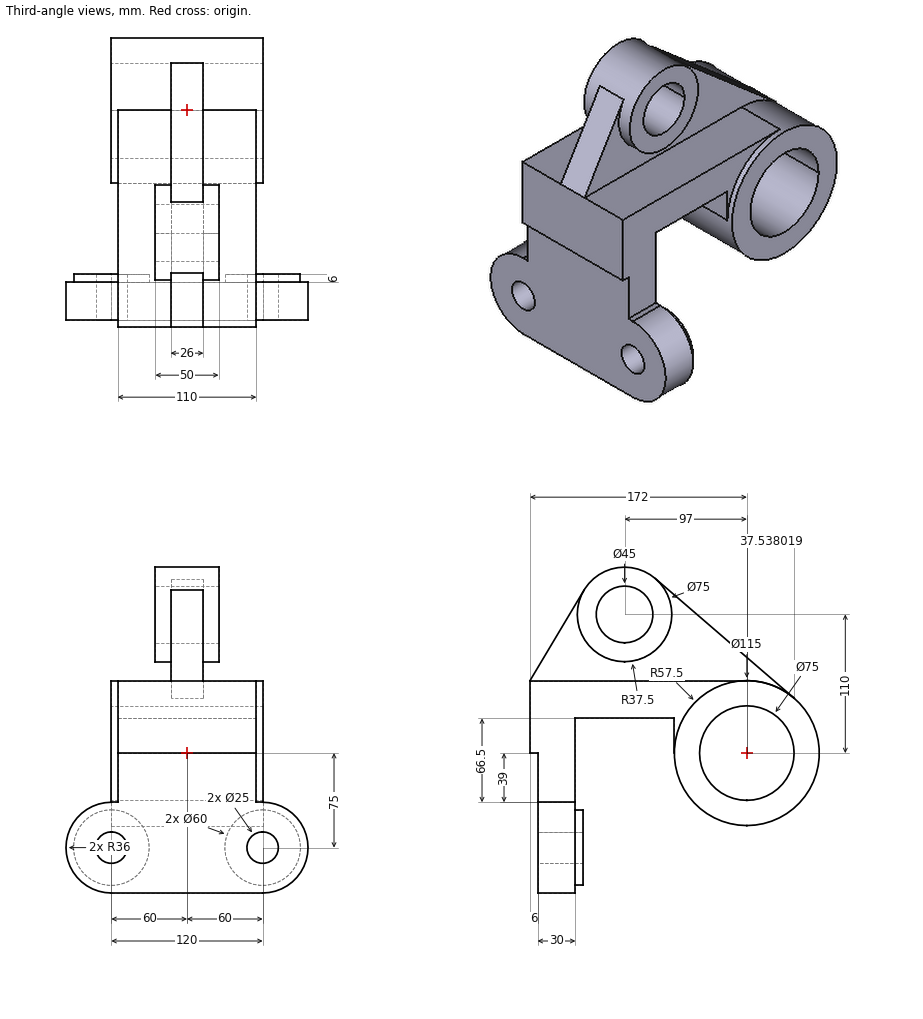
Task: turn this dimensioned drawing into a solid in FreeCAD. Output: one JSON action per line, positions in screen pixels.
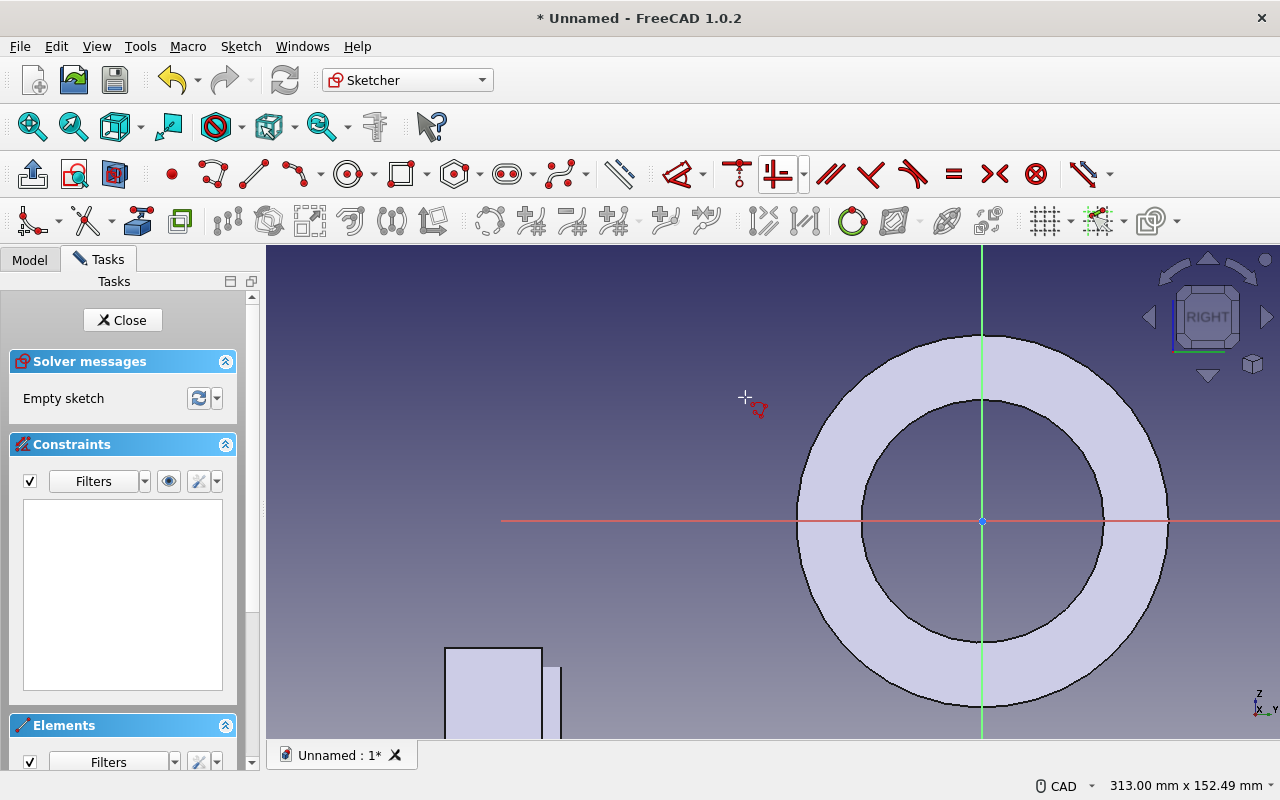
{"action": "left_click", "coordinate": [982, 335]}
{"action": "left_click", "coordinate": [425, 335]}
{"action": "left_click", "coordinate": [425, 521]}
{"action": "left_click", "coordinate": [445, 512]}
{"action": "left_click", "coordinate": [445, 648]}
{"action": "left_click", "coordinate": [542, 648]}
{"action": "left_click", "coordinate": [542, 432]}
{"action": "left_click", "coordinate": [796, 432]}
{"action": "left_click", "coordinate": [796, 521]}
{"action": "right_click", "coordinate": [796, 521]}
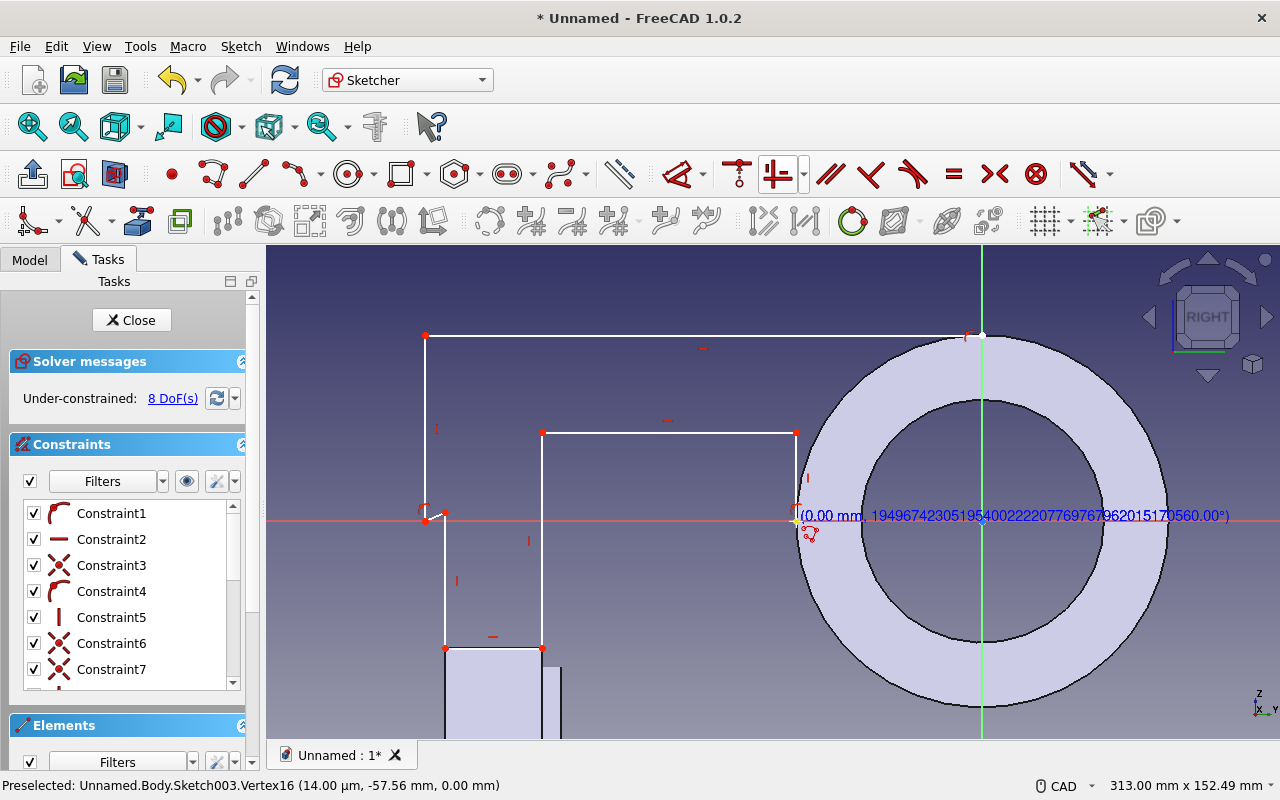
{"action": "key", "text": "g 3 a"}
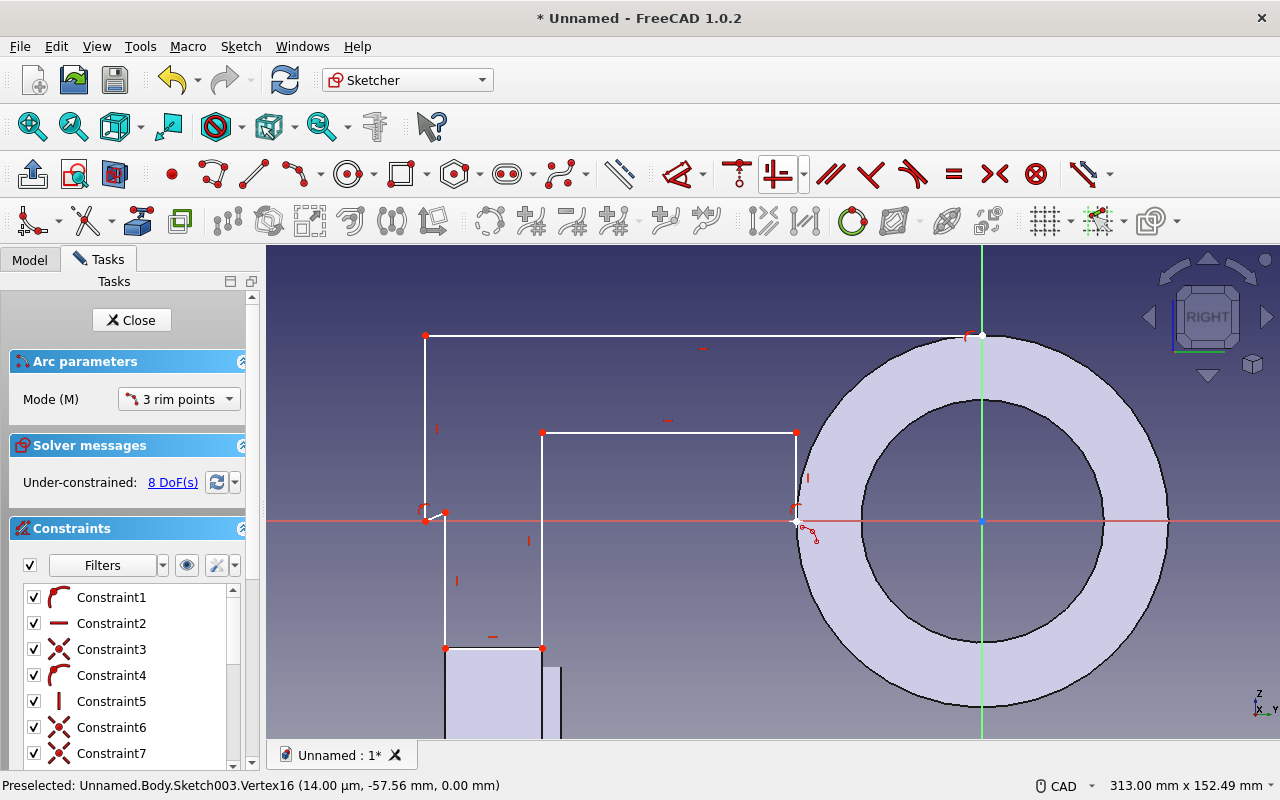
{"action": "left_click", "coordinate": [796, 521]}
{"action": "left_click", "coordinate": [982, 336]}
{"action": "left_click", "coordinate": [851, 389]}
{"action": "key", "text": "Escape"}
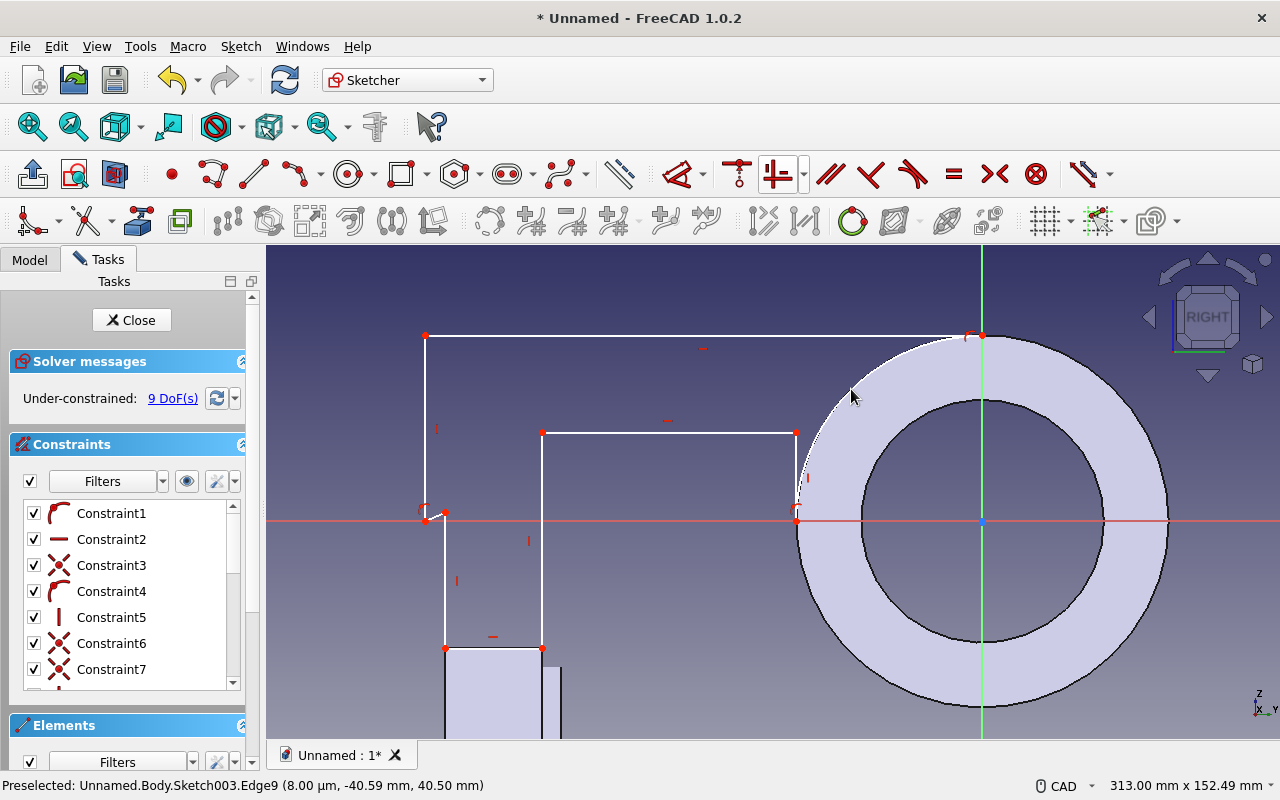
{"action": "scroll", "coordinate": [433, 518], "scroll_direction": "up", "scroll_amount": 3}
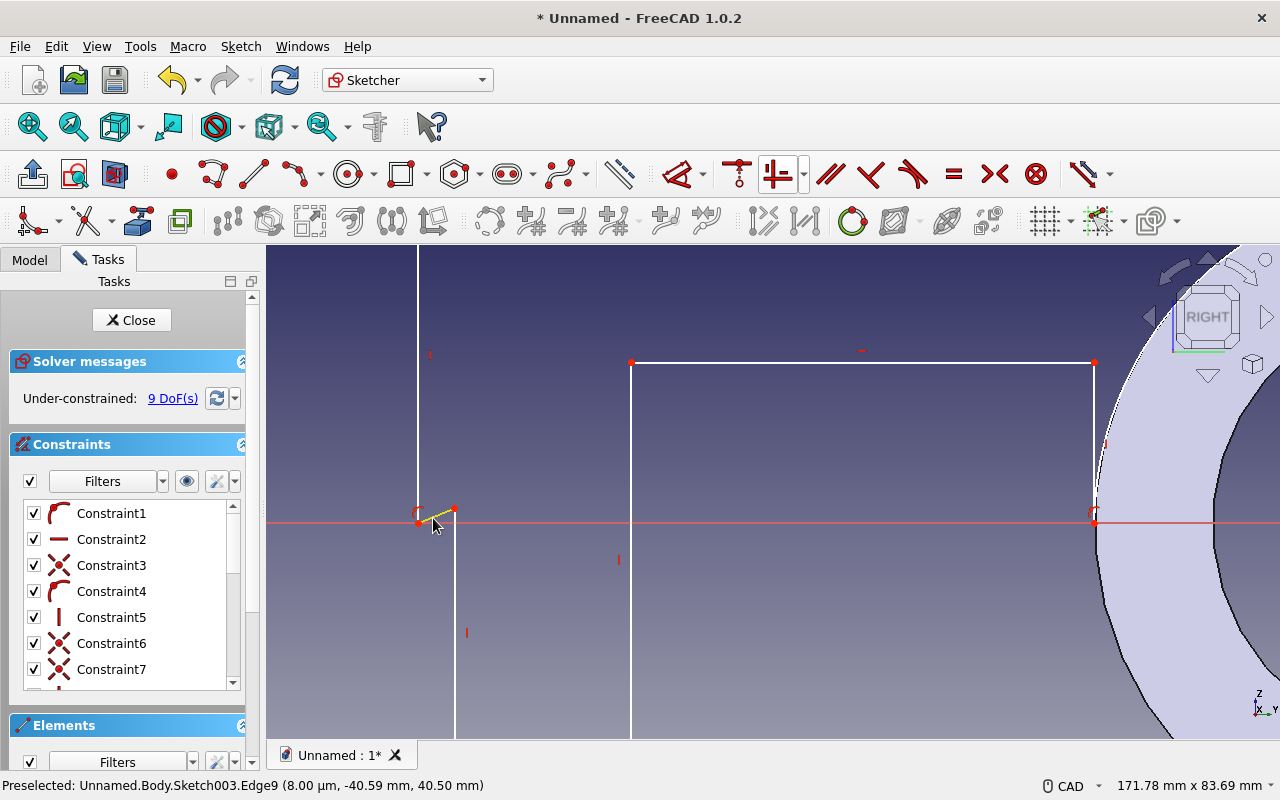
{"action": "left_click", "coordinate": [433, 517]}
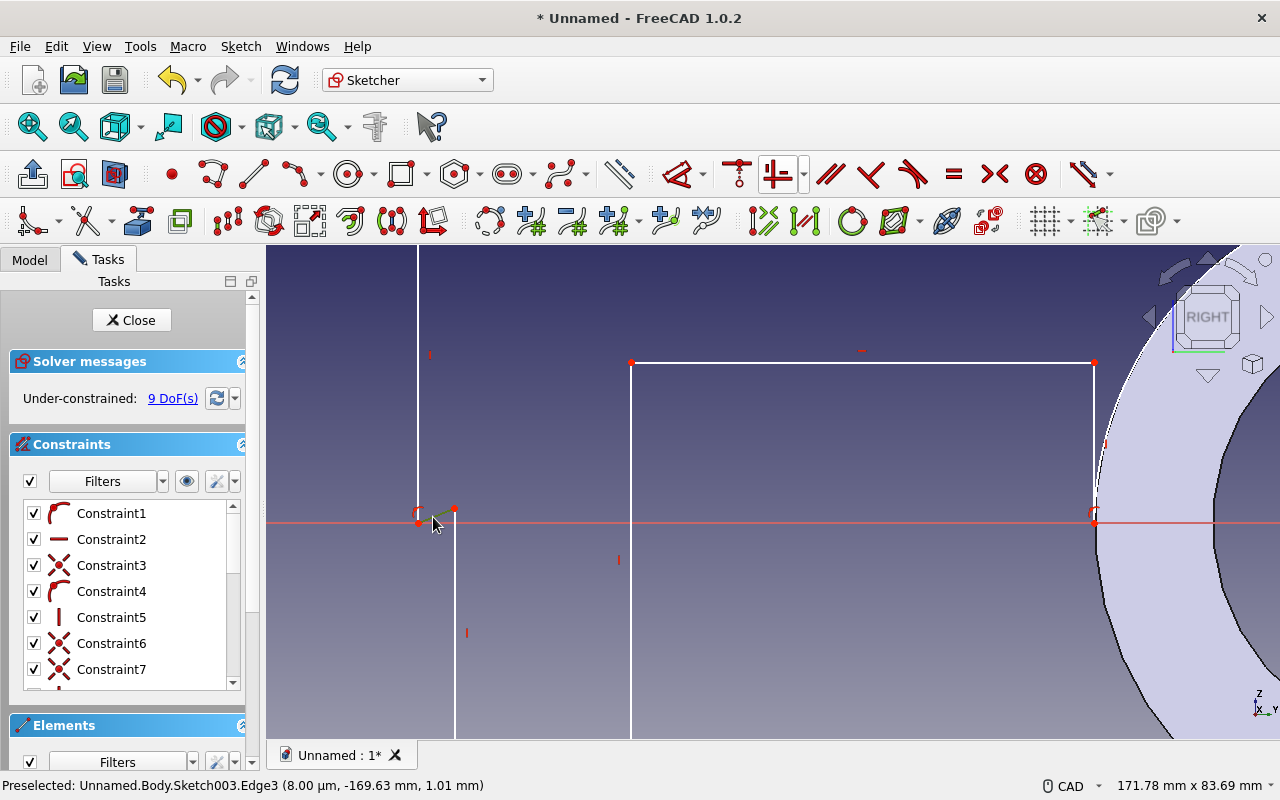
{"action": "key", "text": "h"}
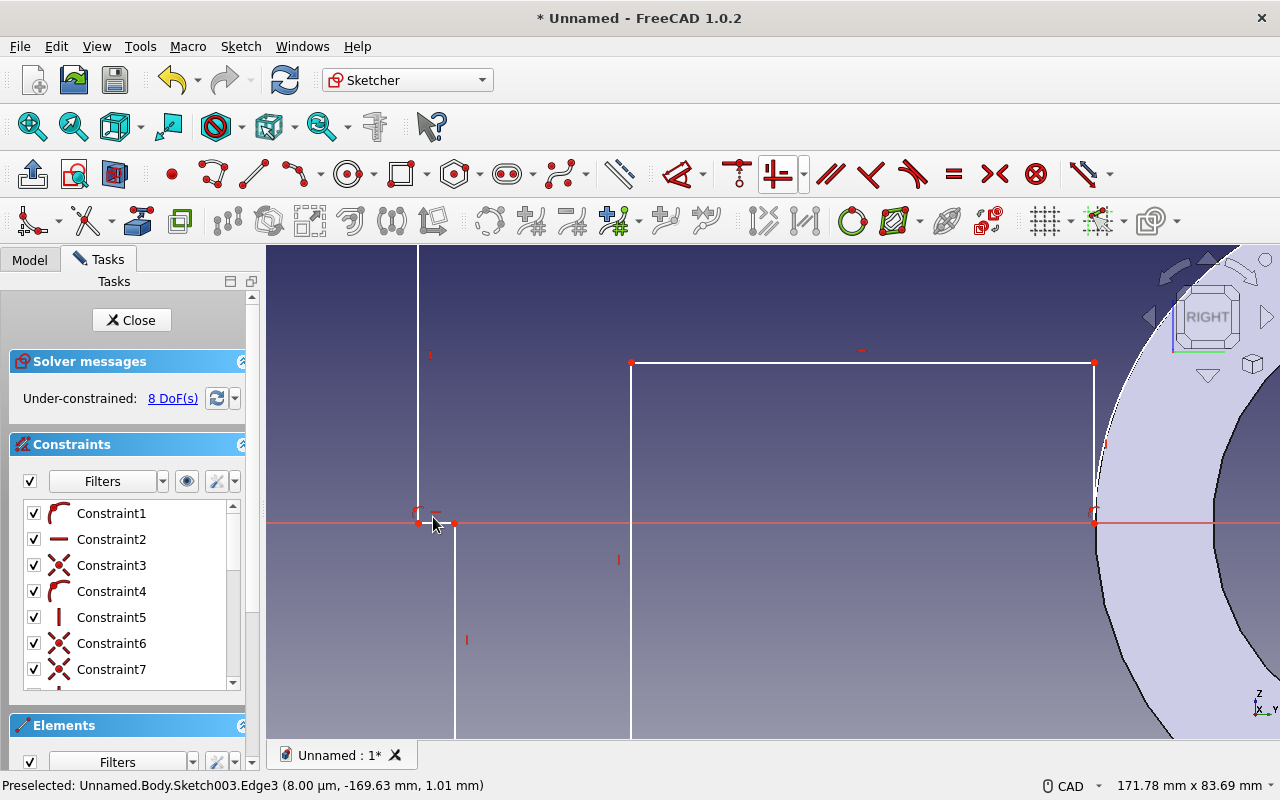
{"action": "scroll", "coordinate": [435, 520], "scroll_direction": "down", "scroll_amount": 3}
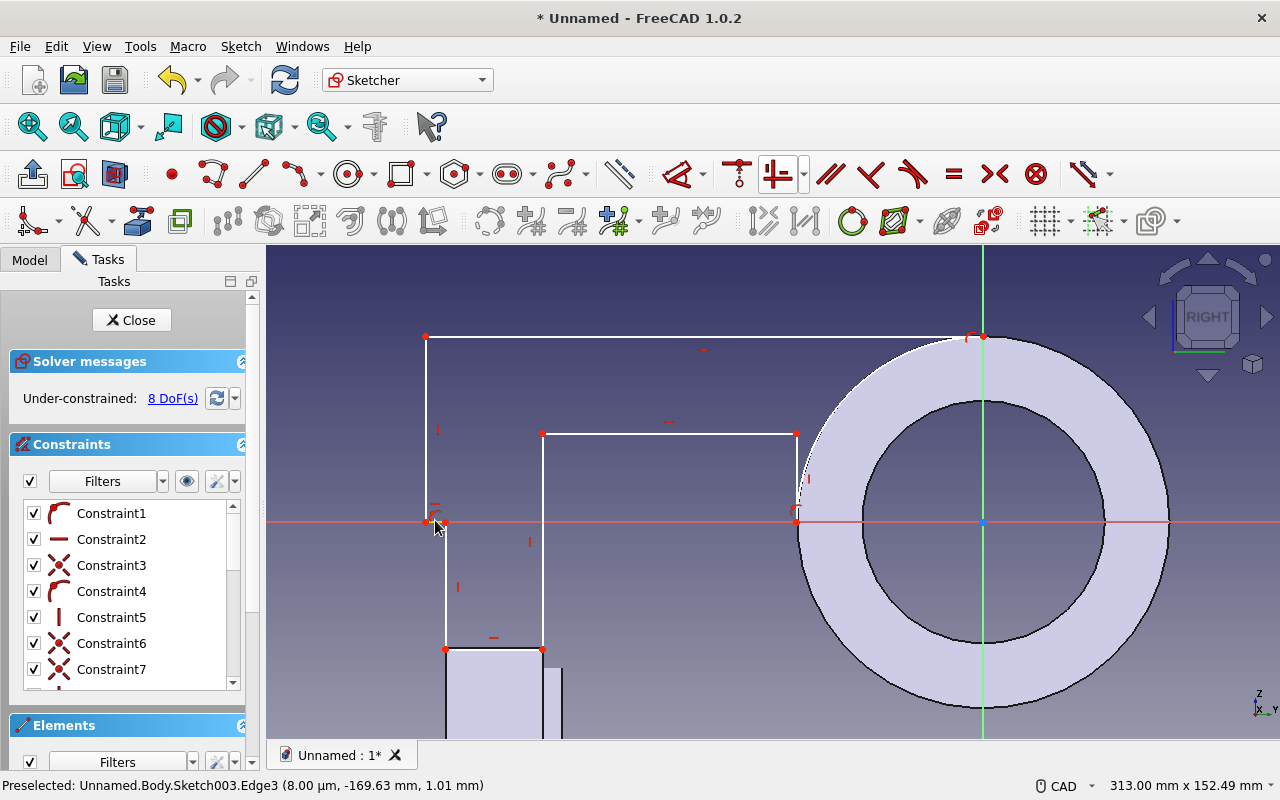
{"action": "left_click_drag", "start_coordinate": [973, 512], "coordinate": [993, 533]}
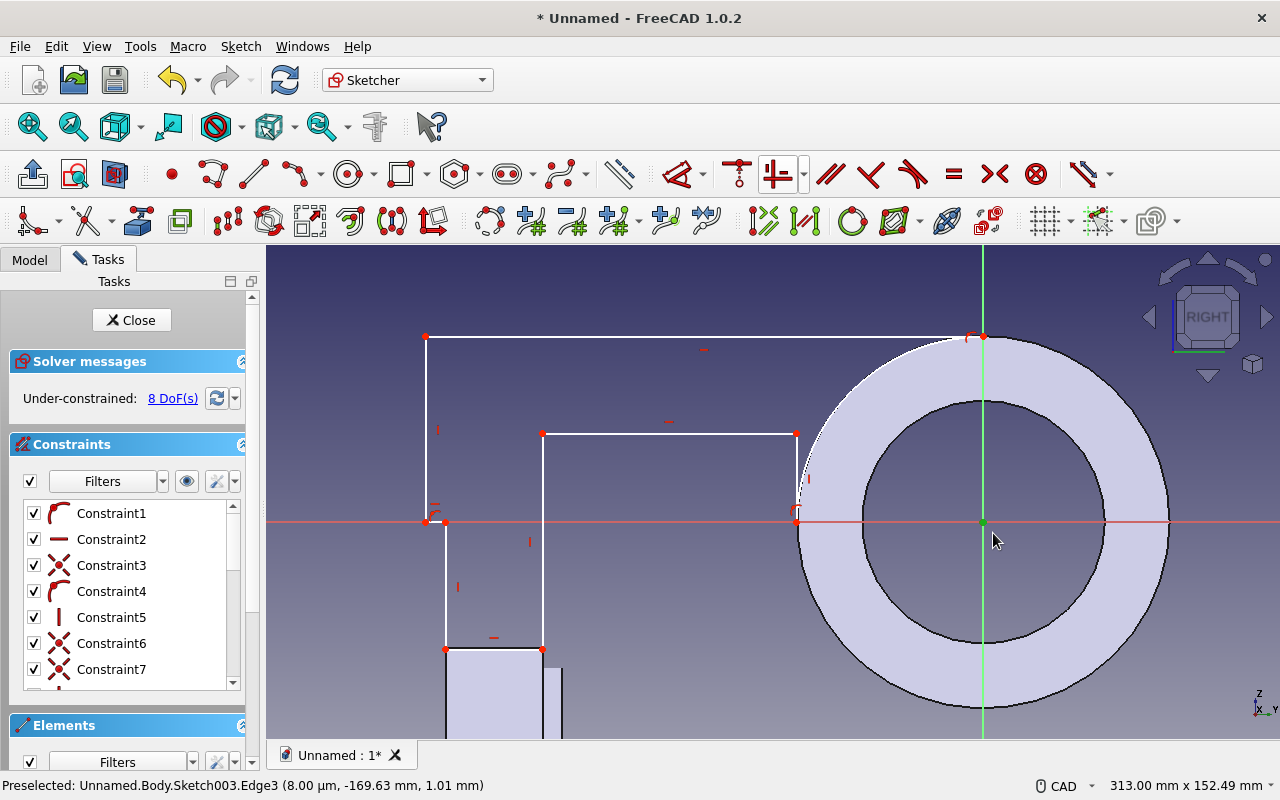
{"action": "key", "text": "c"}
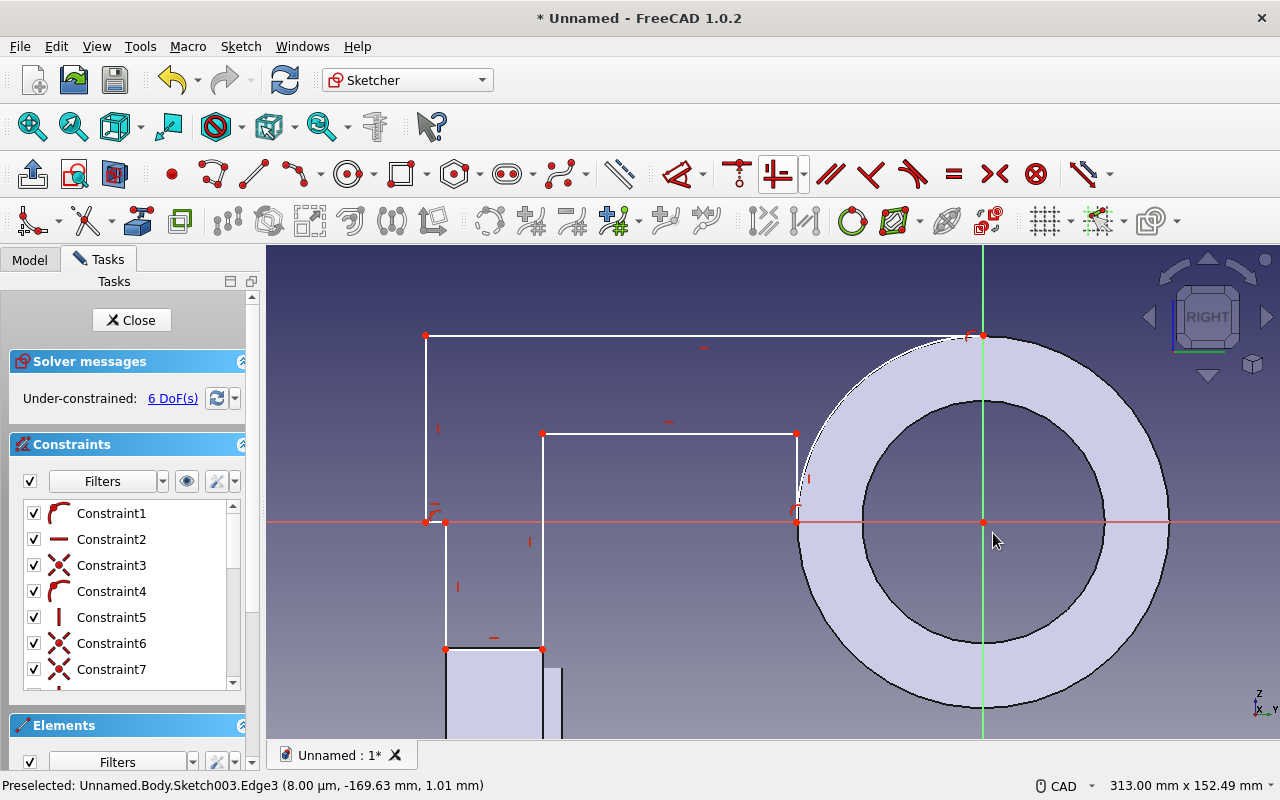
{"action": "key", "text": "d"}